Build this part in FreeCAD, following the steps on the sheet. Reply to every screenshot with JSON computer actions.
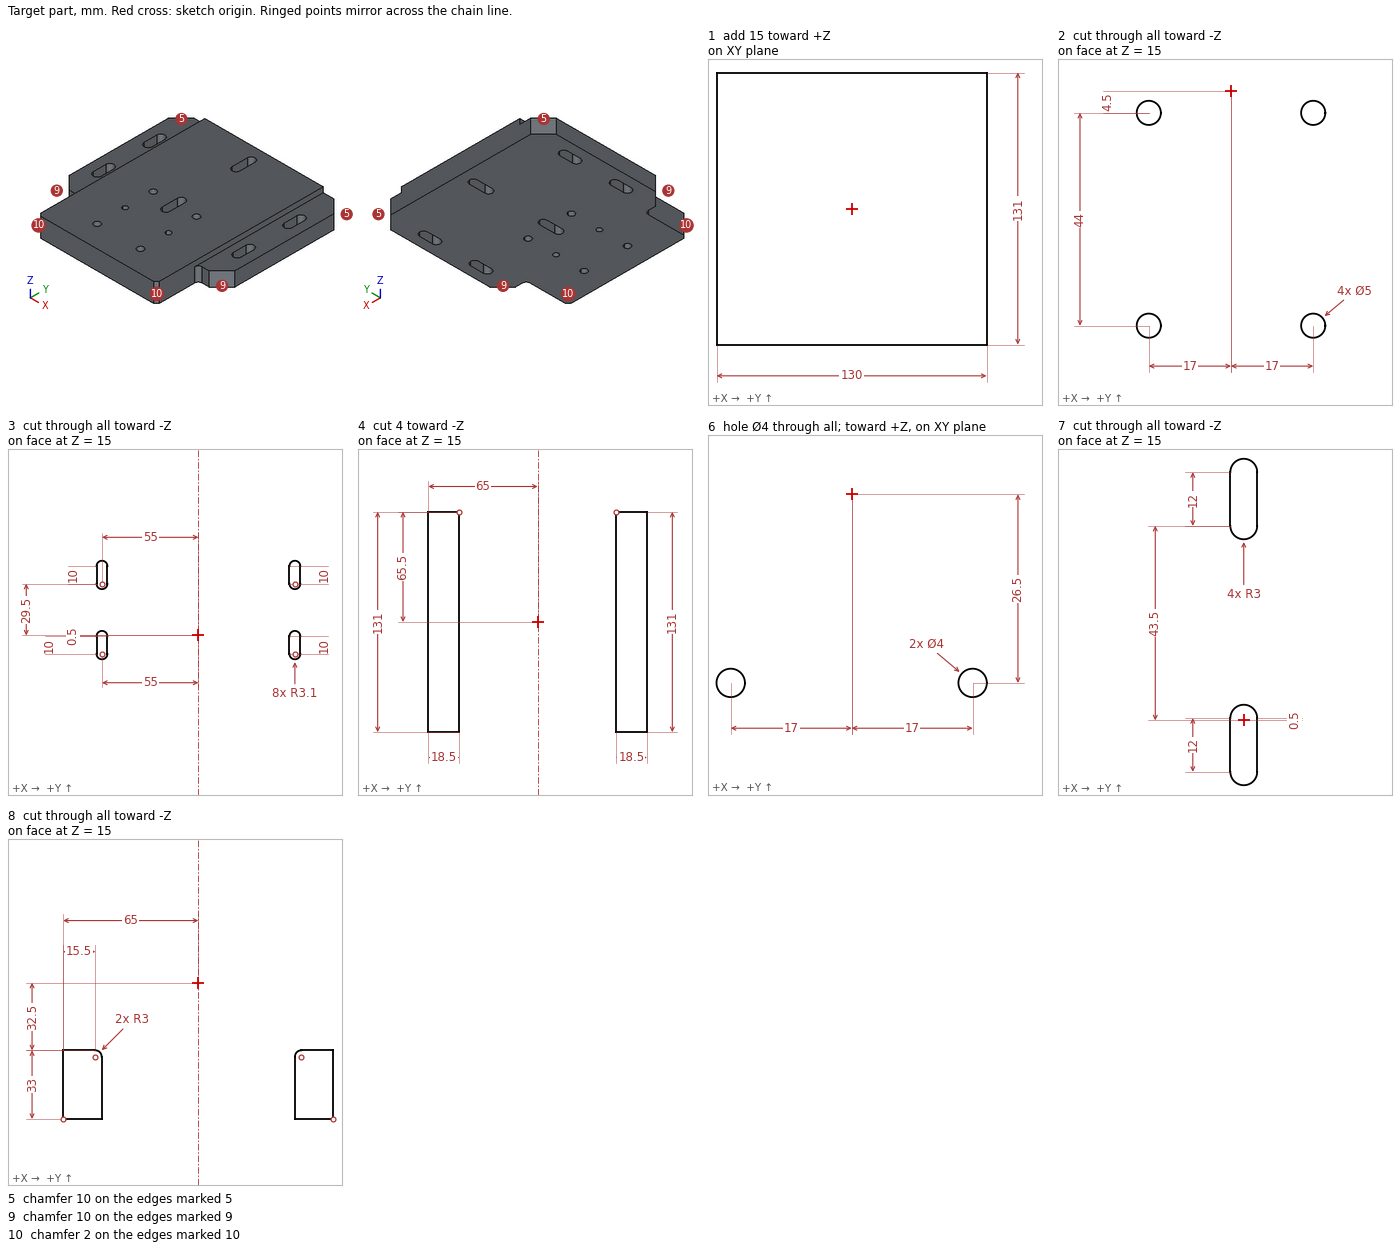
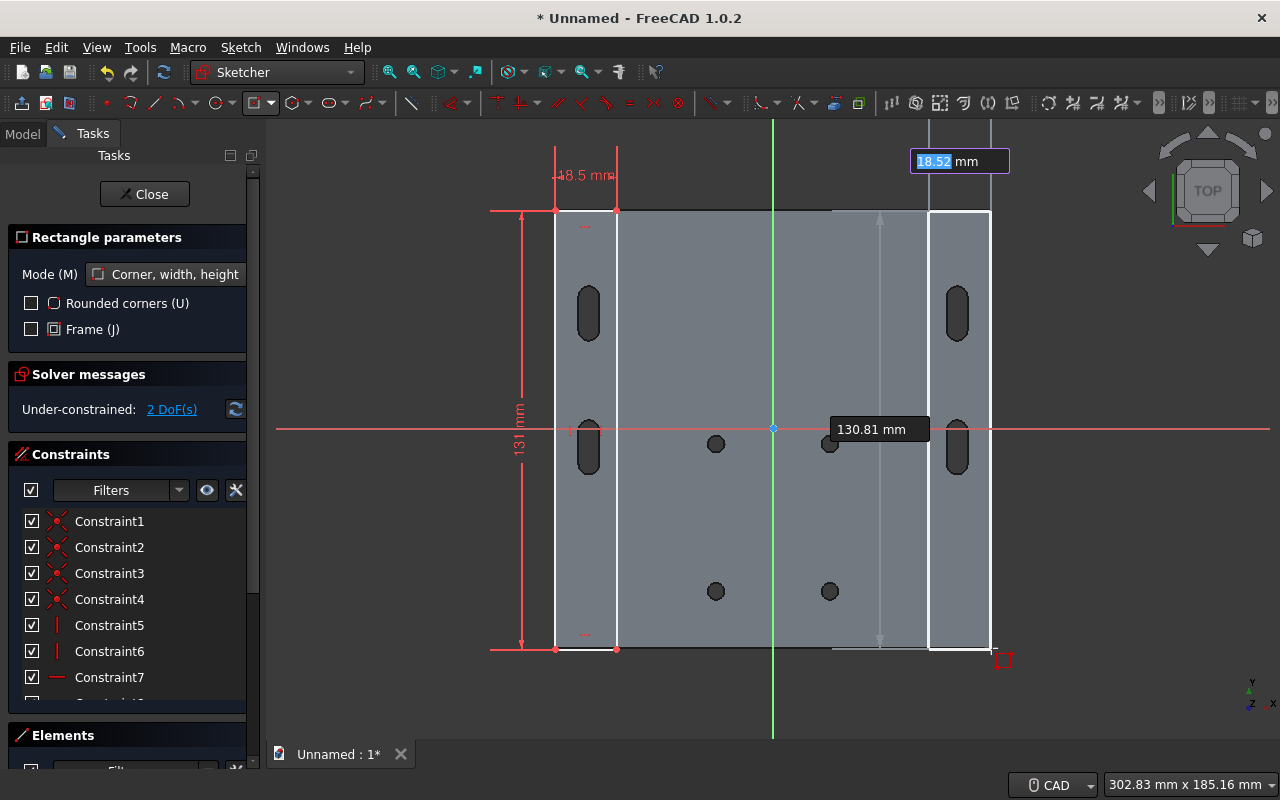
{"action": "type", "text": "18.5"}
{"action": "key", "text": "Tab"}
{"action": "type", "text": "131"}
{"action": "key", "text": "Return"}
{"action": "key", "text": "Escape"}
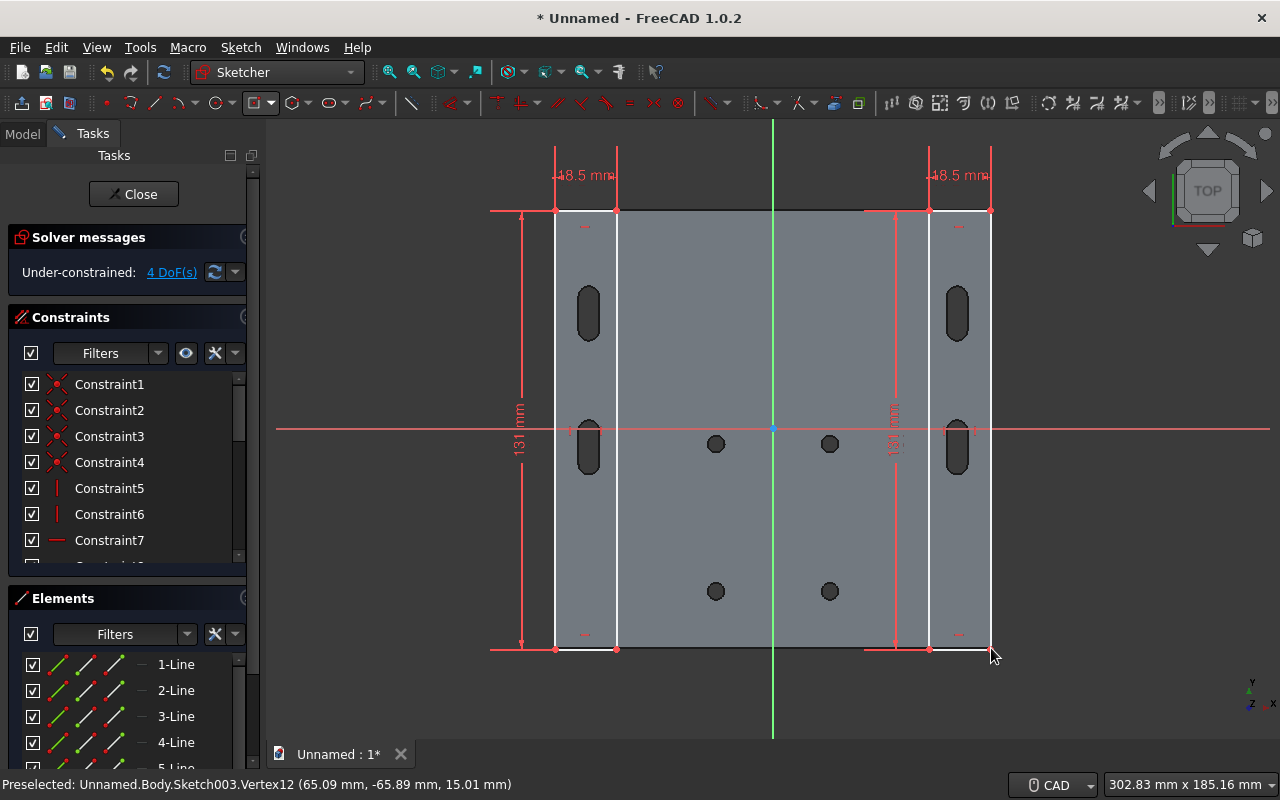
{"action": "left_click", "coordinate": [617, 211]}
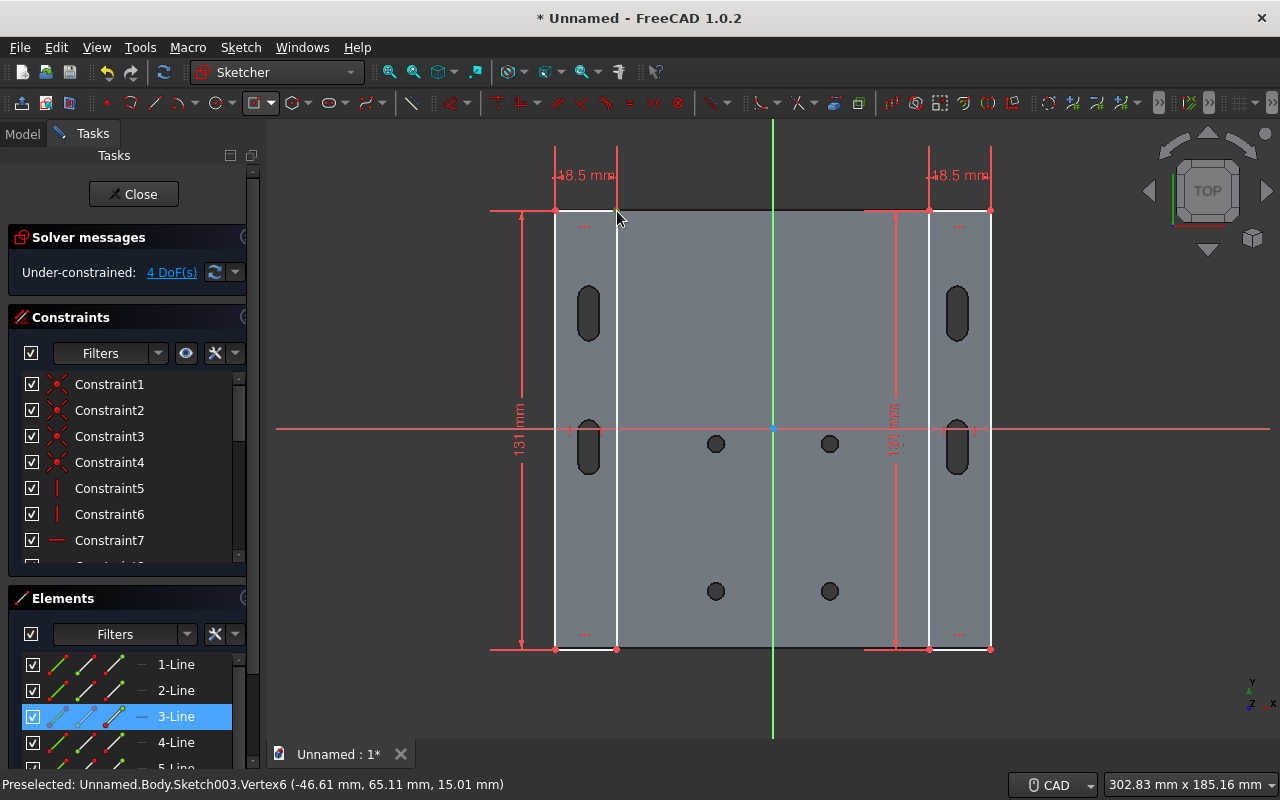
{"action": "left_click", "coordinate": [929, 211]}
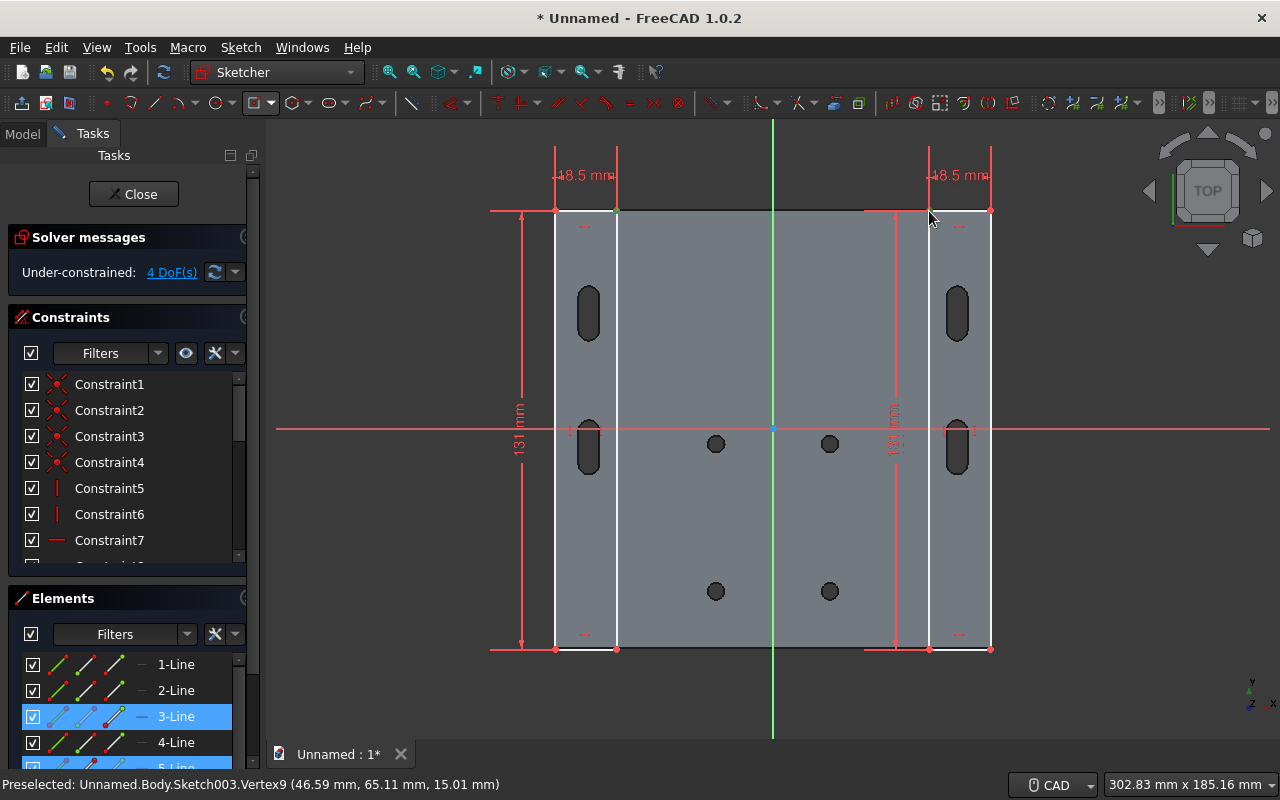
{"action": "left_click", "coordinate": [773, 671]}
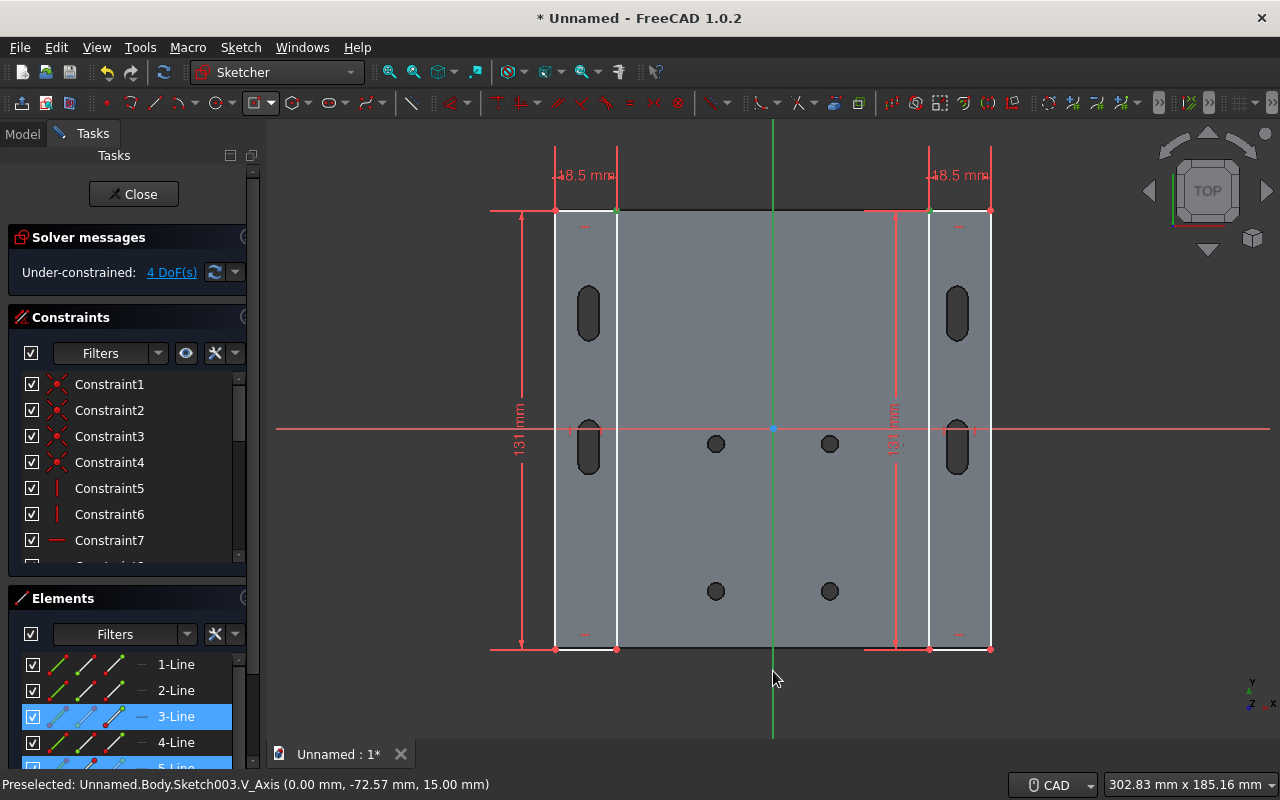
{"action": "key", "text": "s"}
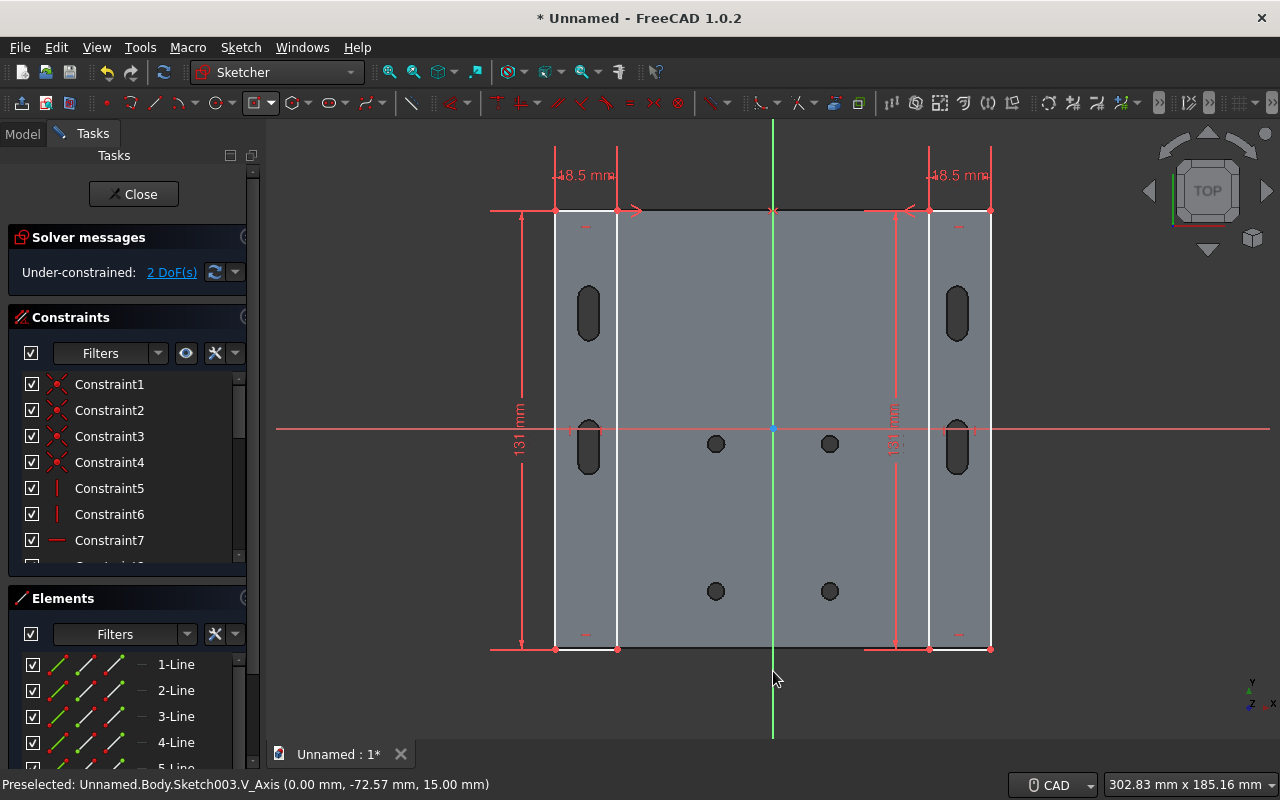
{"action": "key", "text": "d"}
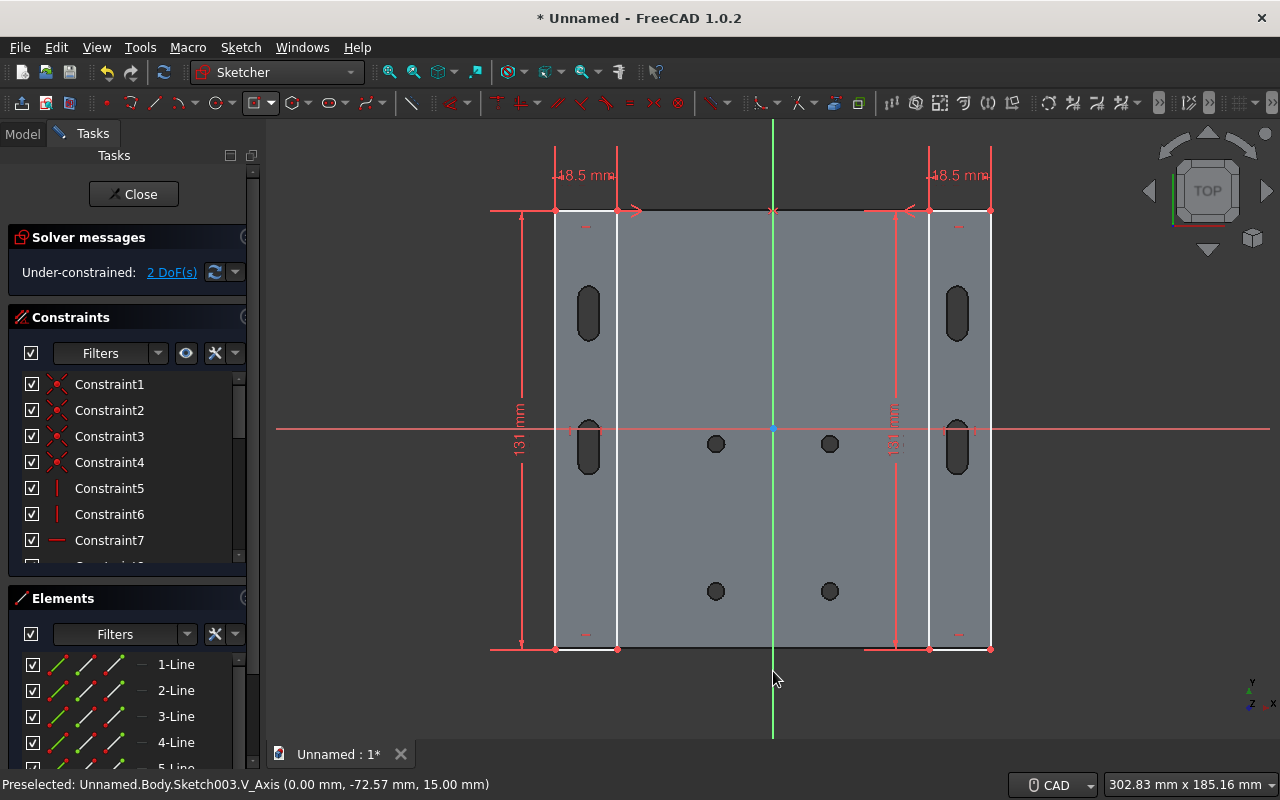
{"action": "left_click", "coordinate": [555, 211]}
{"action": "left_click", "coordinate": [664, 177]}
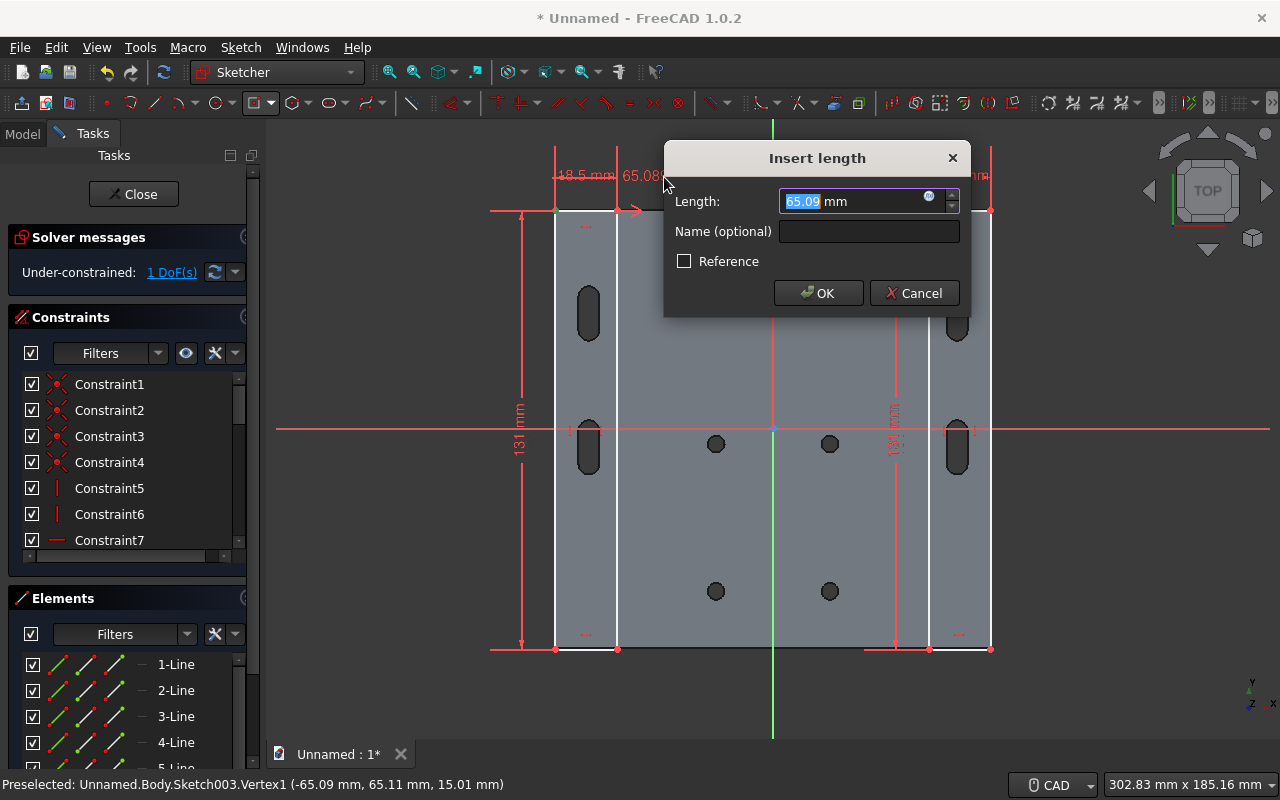
{"action": "type", "text": "65"}
{"action": "key", "text": "Return"}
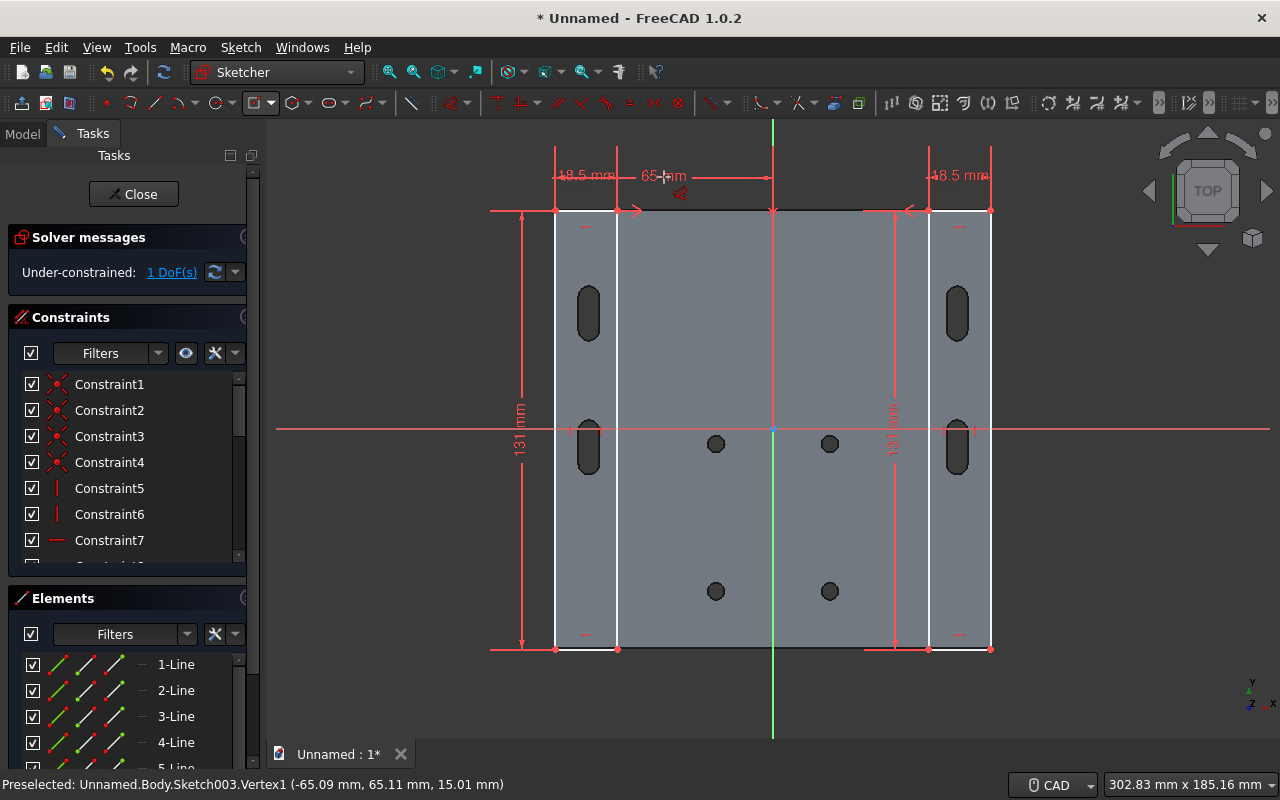
{"action": "left_click", "coordinate": [555, 211]}
{"action": "left_click", "coordinate": [521, 320]}